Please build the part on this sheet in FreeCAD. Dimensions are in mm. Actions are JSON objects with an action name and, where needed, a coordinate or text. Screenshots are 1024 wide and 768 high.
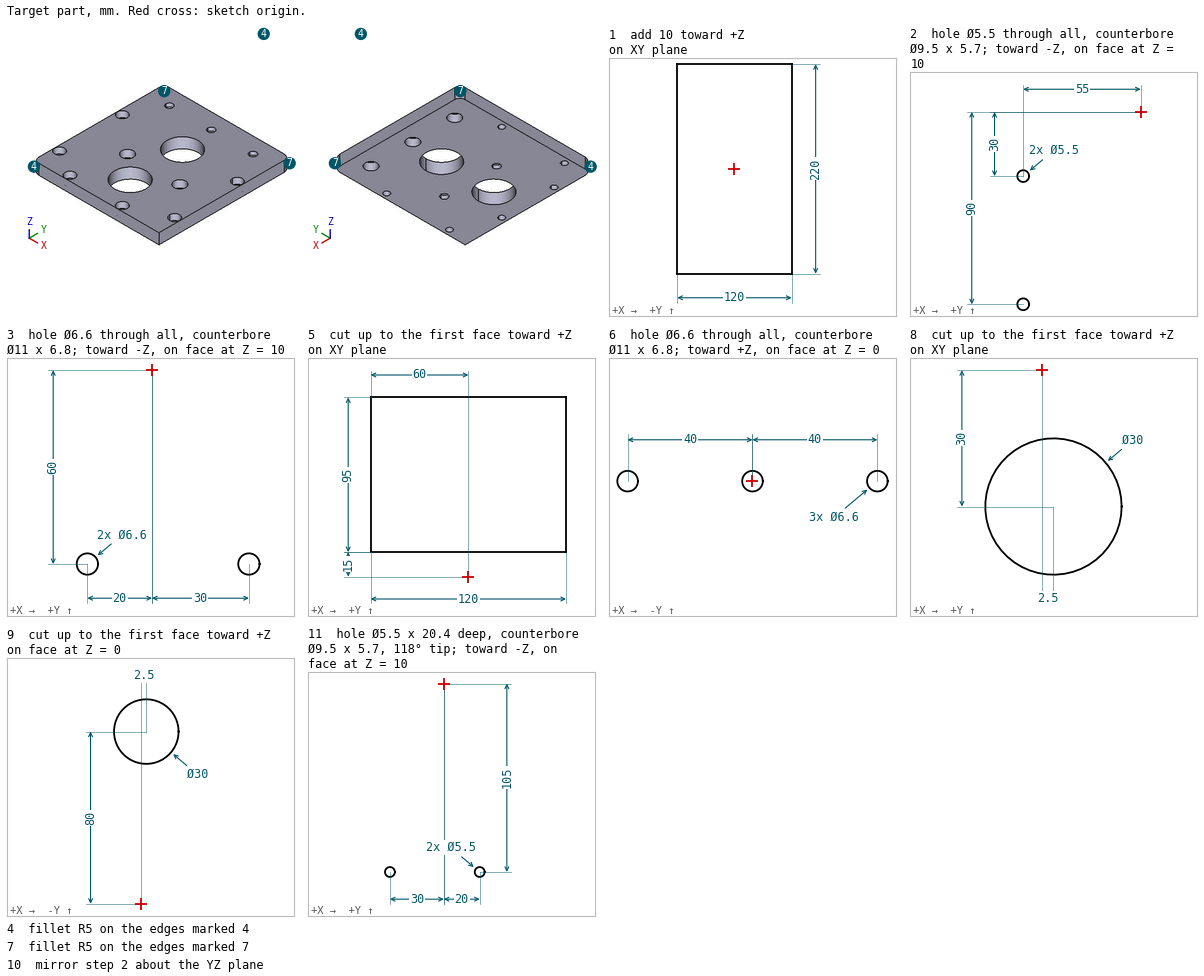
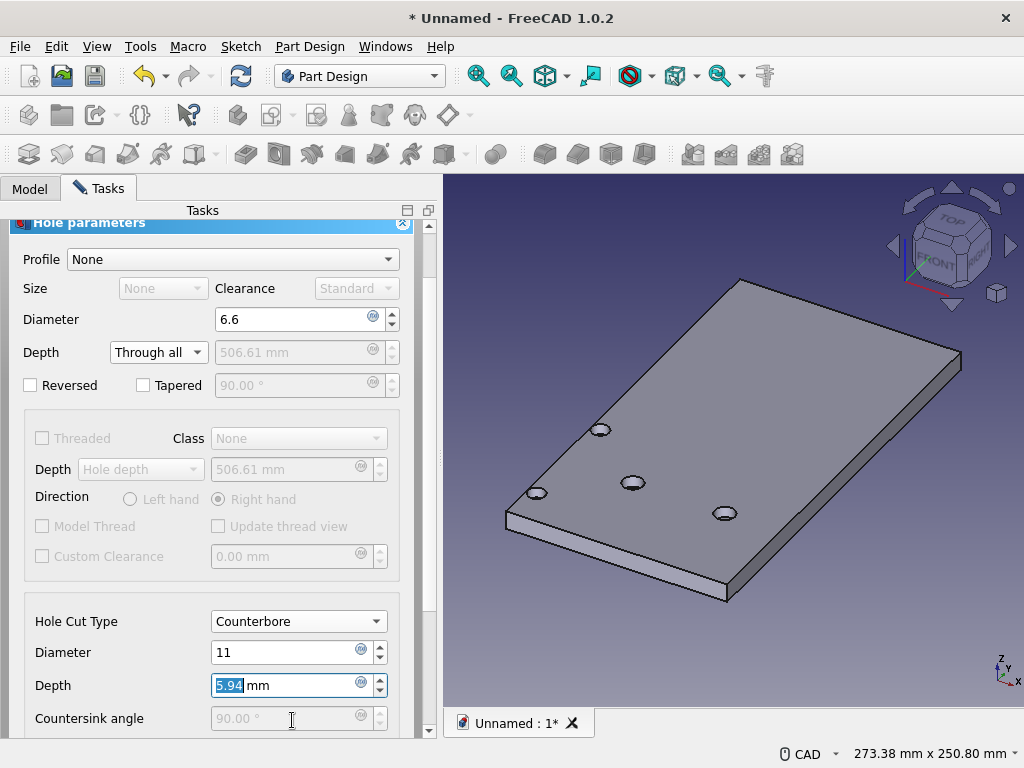
{"action": "type", "text": "6.8"}
{"action": "key", "text": "Tab"}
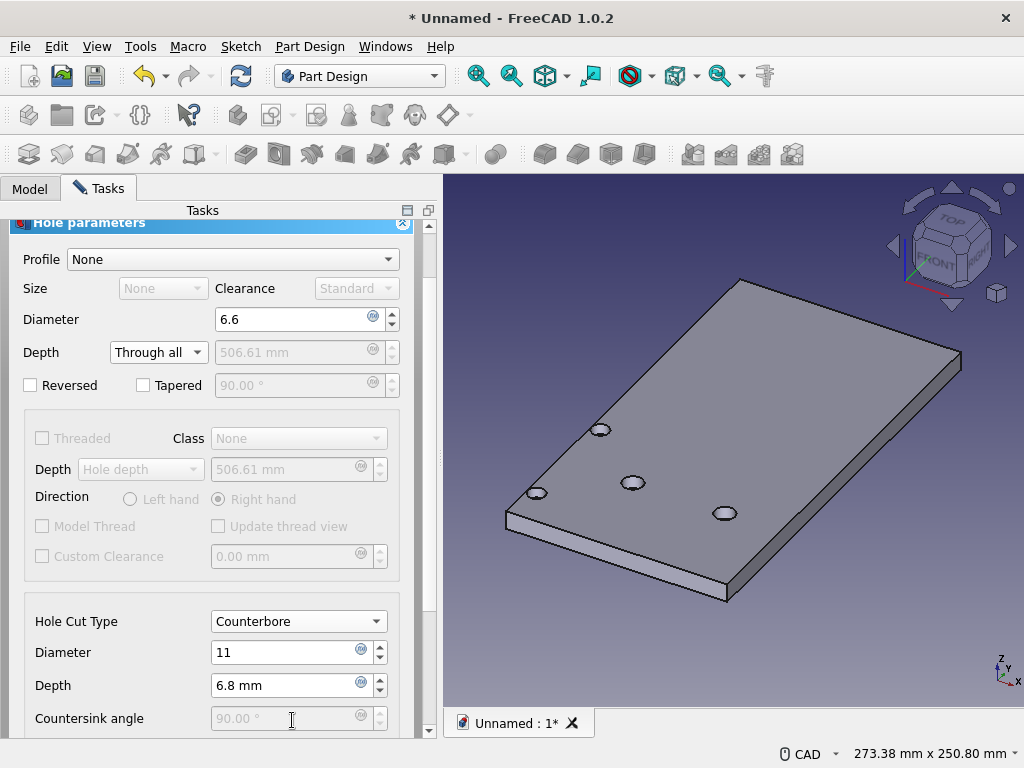
{"action": "scroll", "coordinate": [429, 479], "scroll_direction": "up", "scroll_amount": 2}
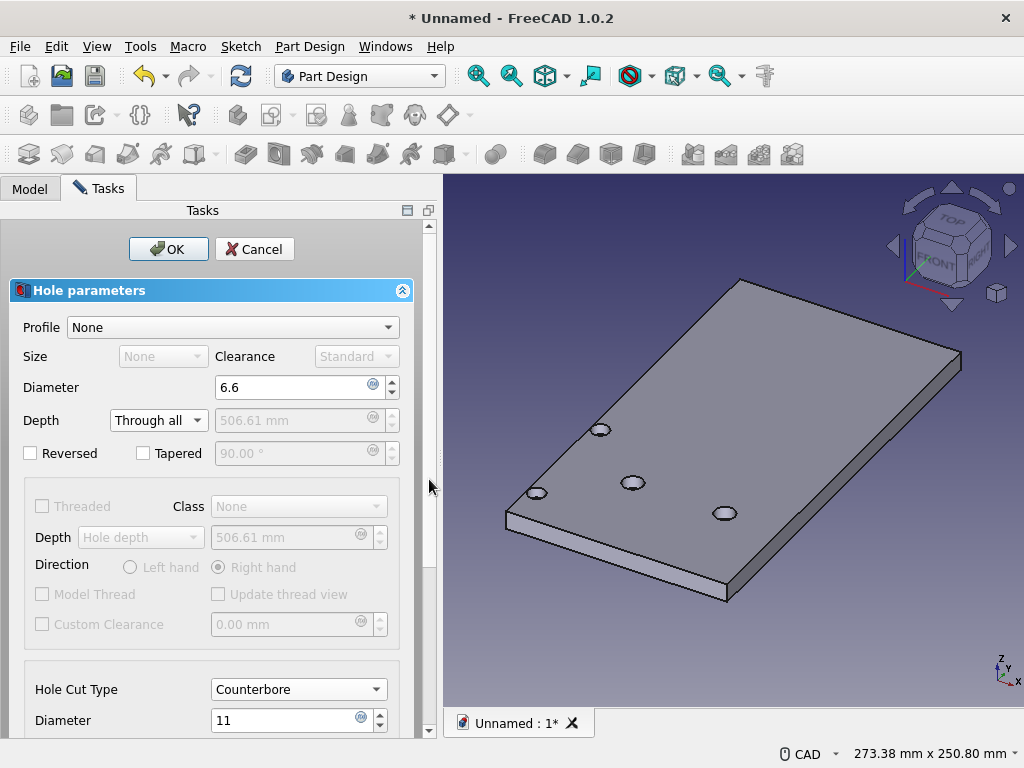
{"action": "left_click", "coordinate": [169, 249]}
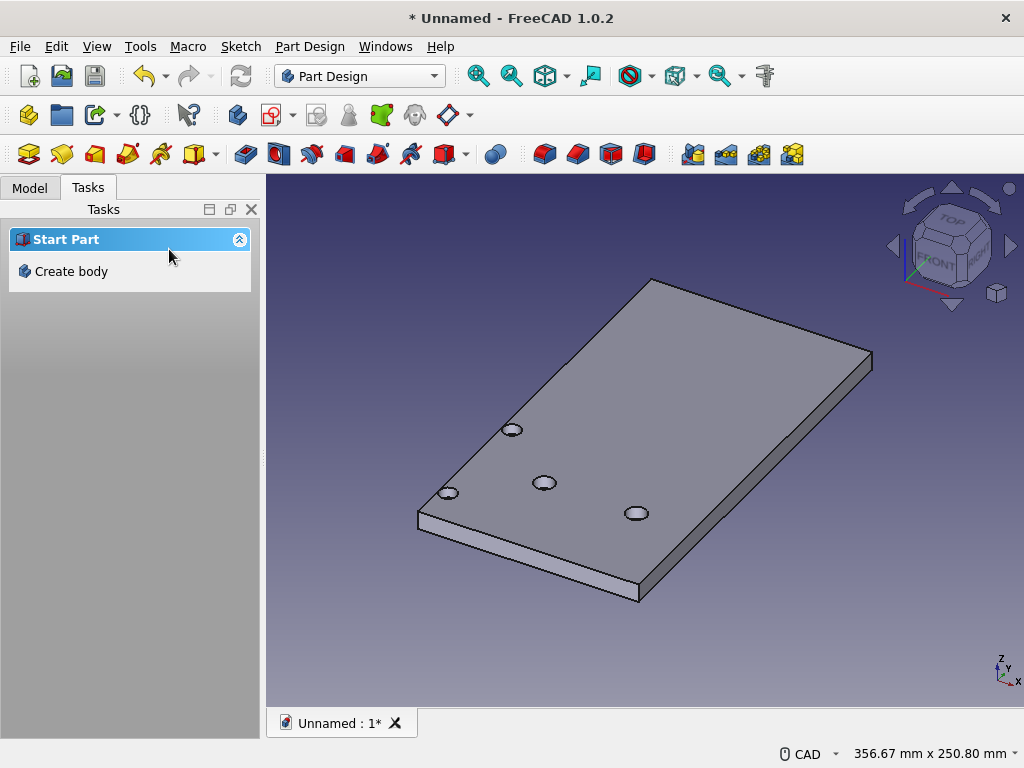
{"action": "scroll", "coordinate": [651, 287], "scroll_direction": "up", "scroll_amount": 4}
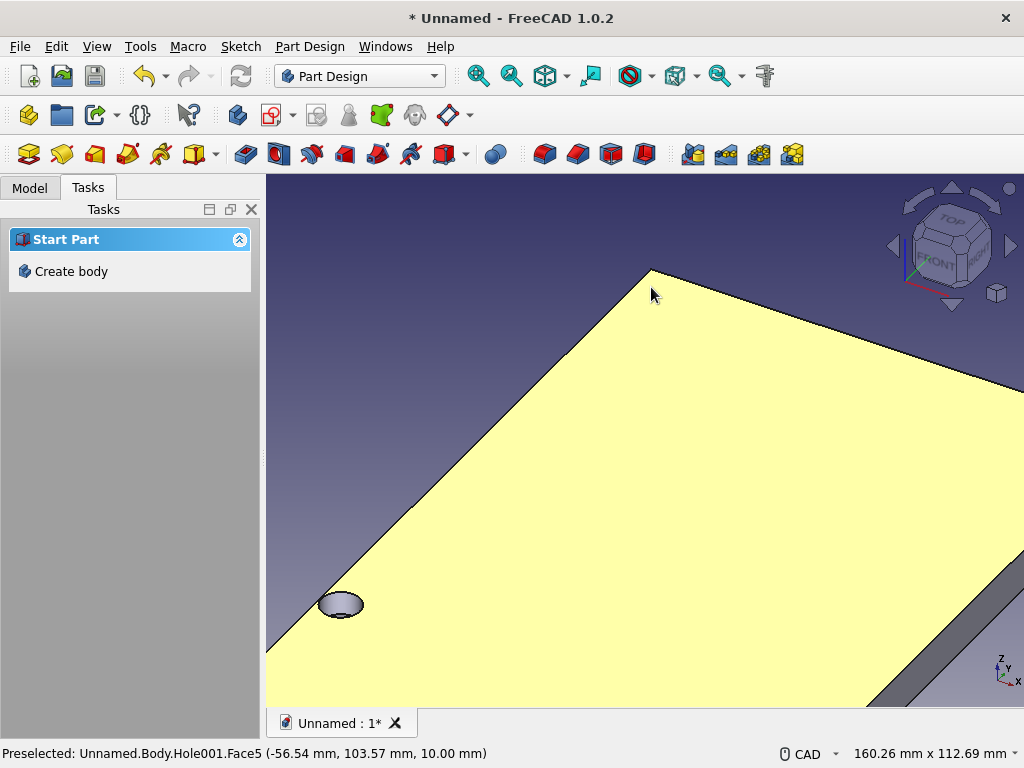
{"action": "key", "text": "v f"}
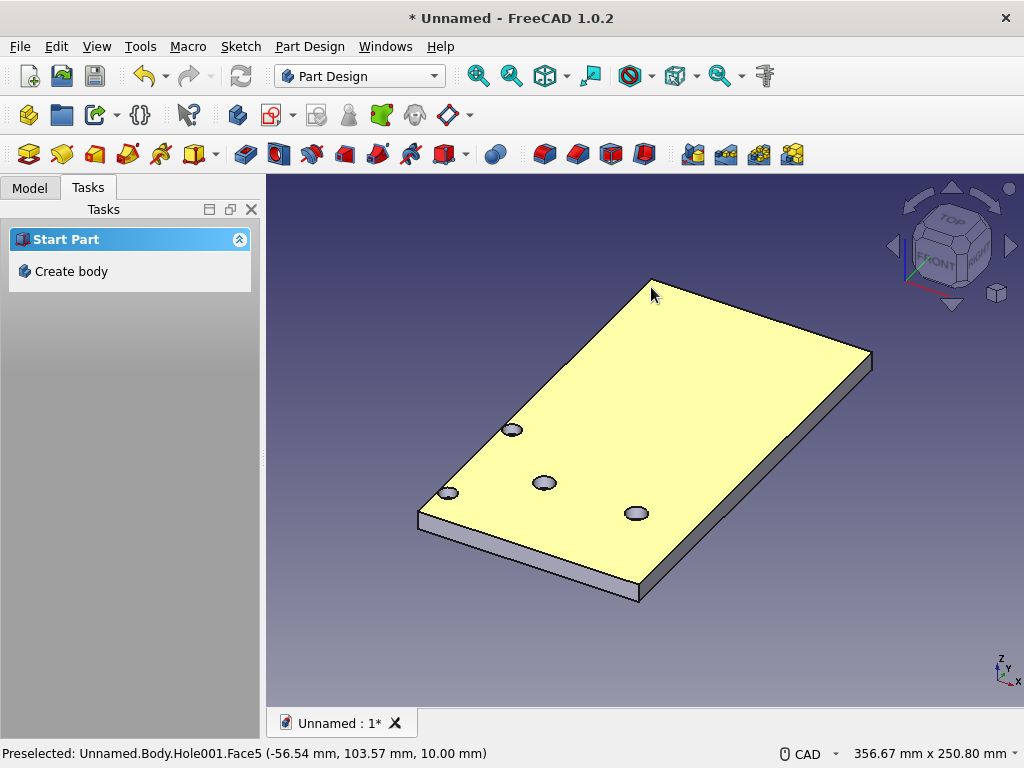
{"action": "key", "text": "0"}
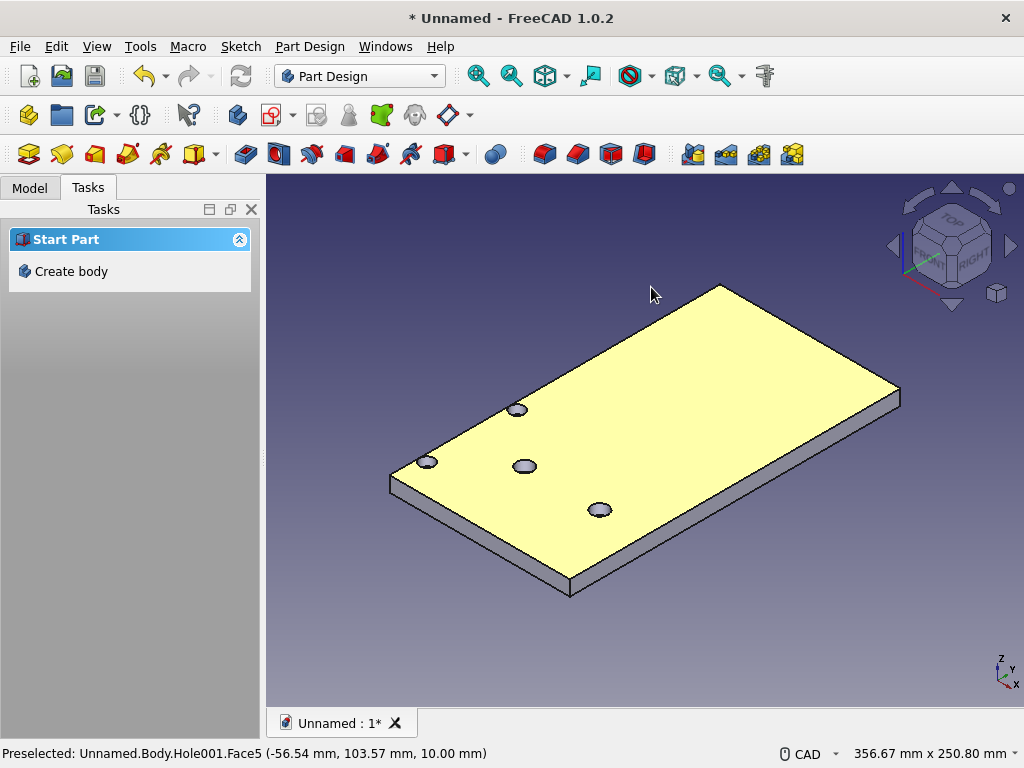
{"action": "scroll", "coordinate": [720, 292], "scroll_direction": "up", "scroll_amount": 4}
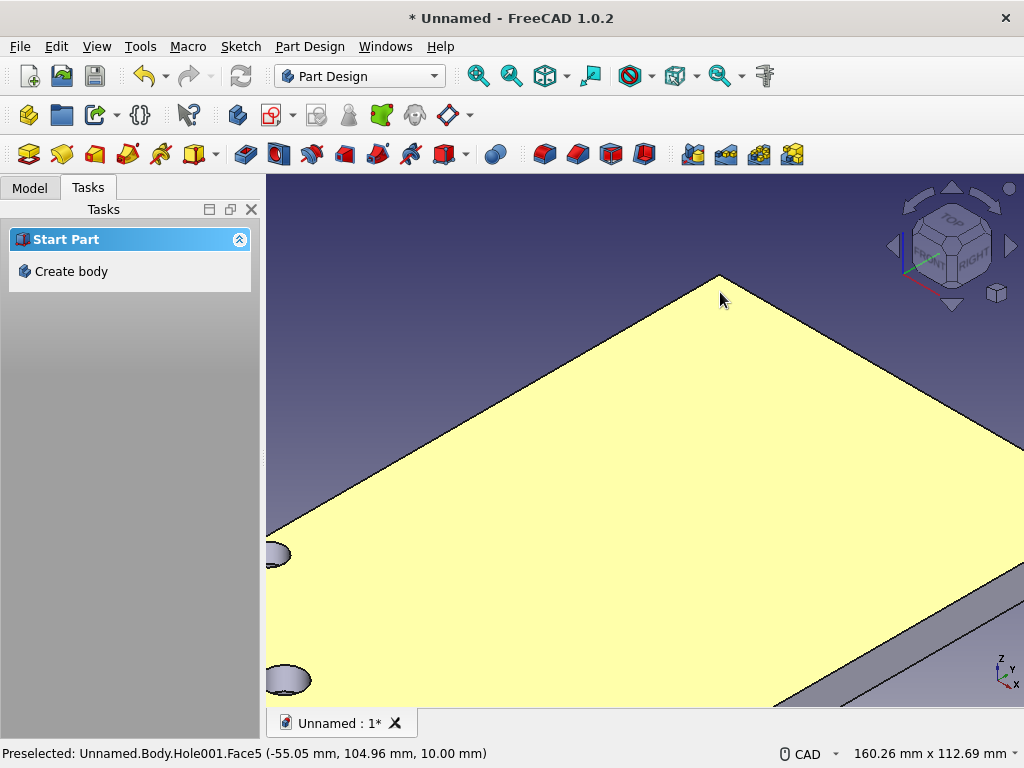
{"action": "key", "text": "v f"}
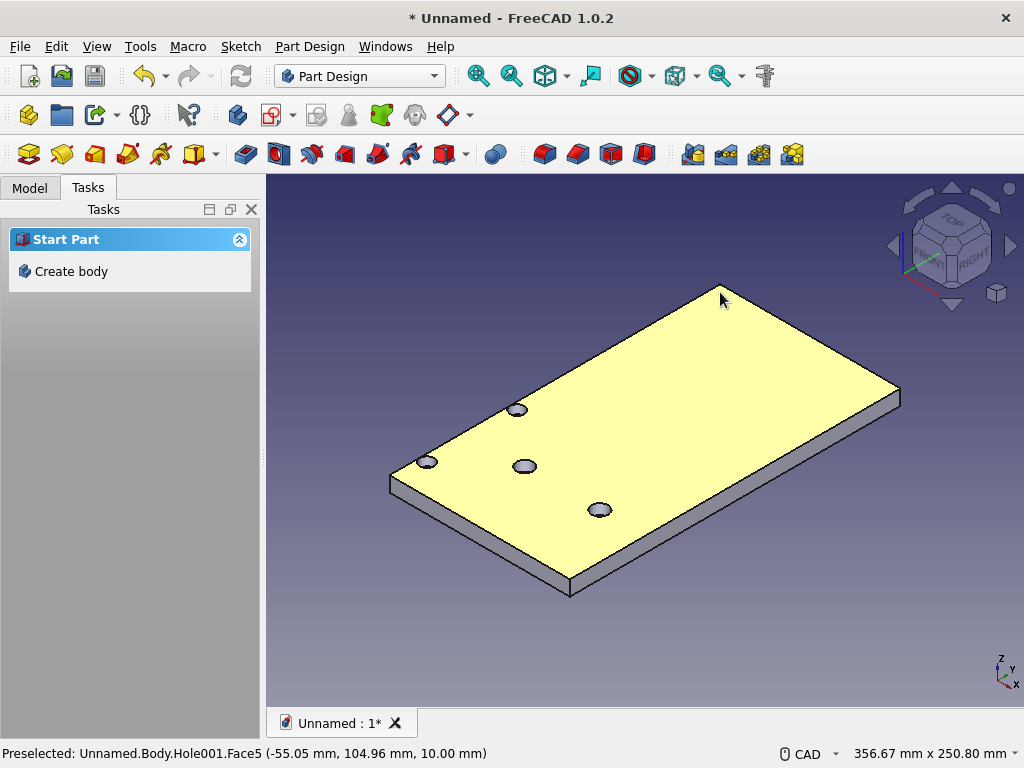
{"action": "key", "text": "2"}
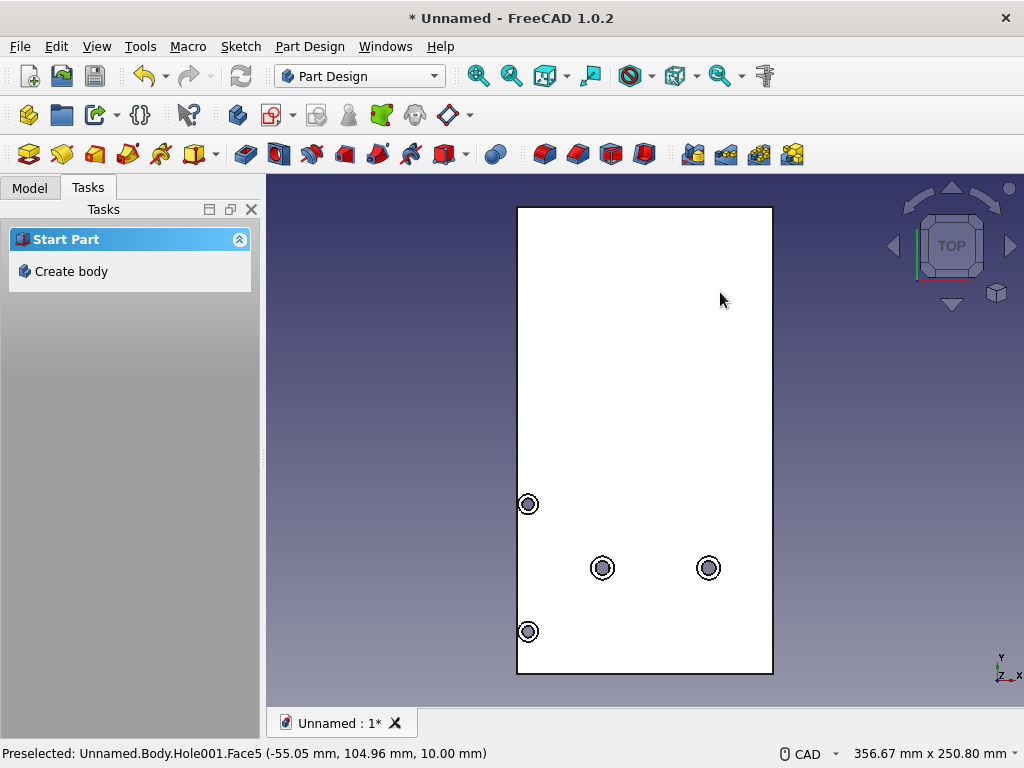
{"action": "scroll", "coordinate": [517, 206], "scroll_direction": "up", "scroll_amount": 4}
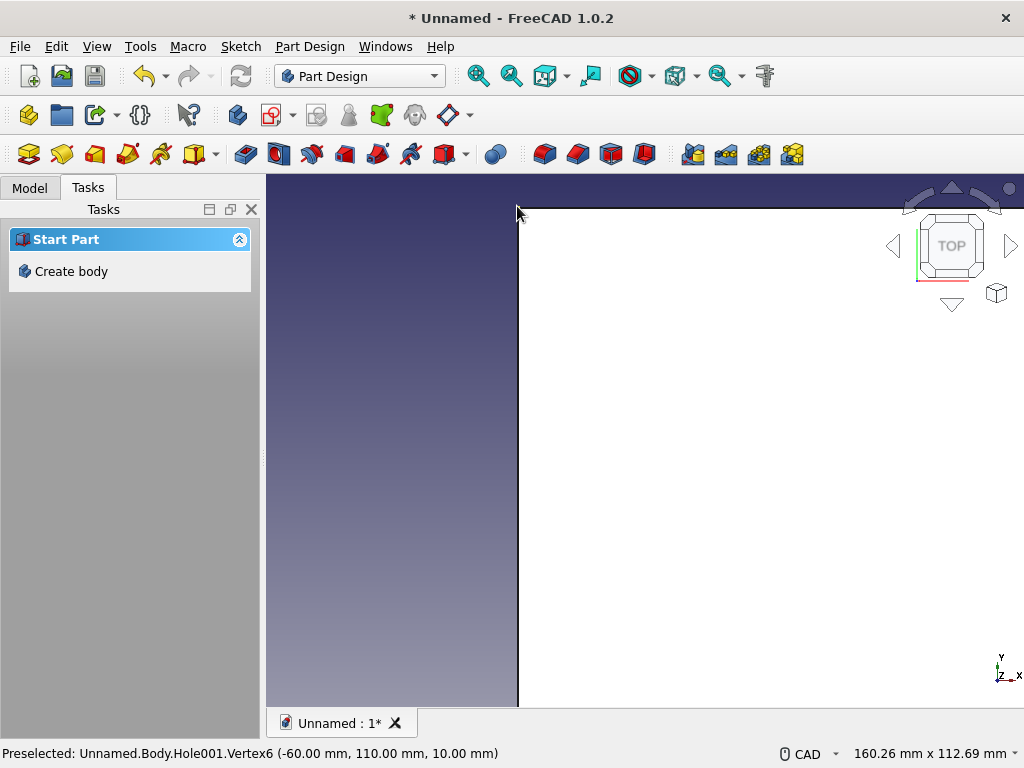
{"action": "key", "text": "v f"}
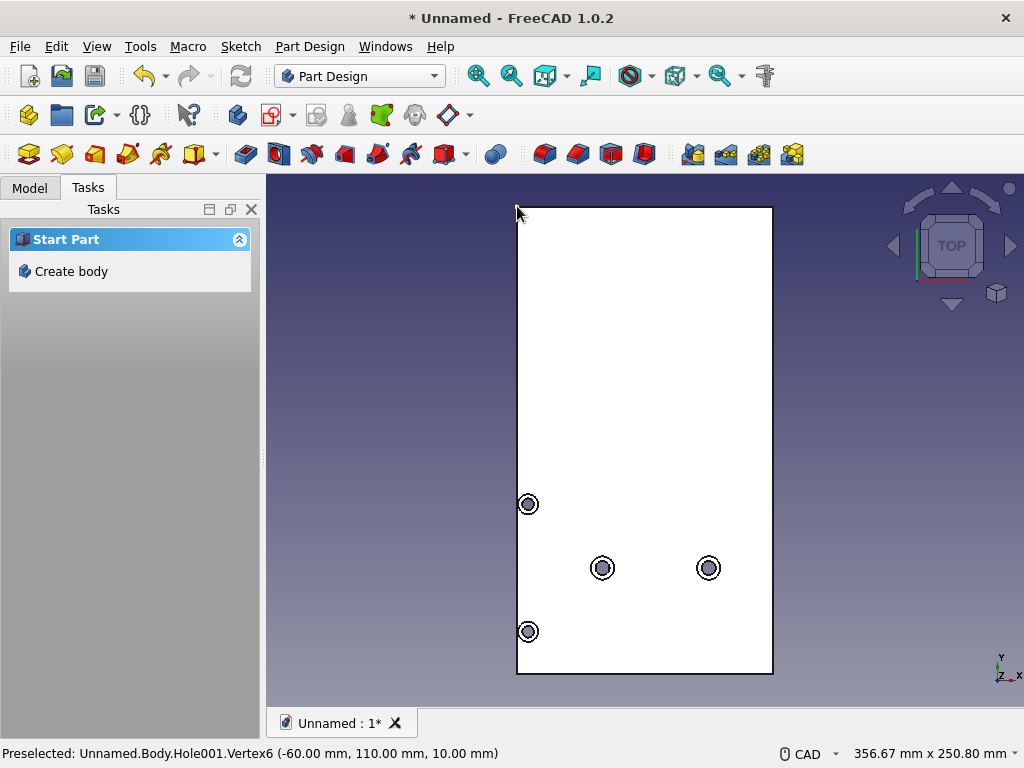
{"action": "key", "text": "1"}